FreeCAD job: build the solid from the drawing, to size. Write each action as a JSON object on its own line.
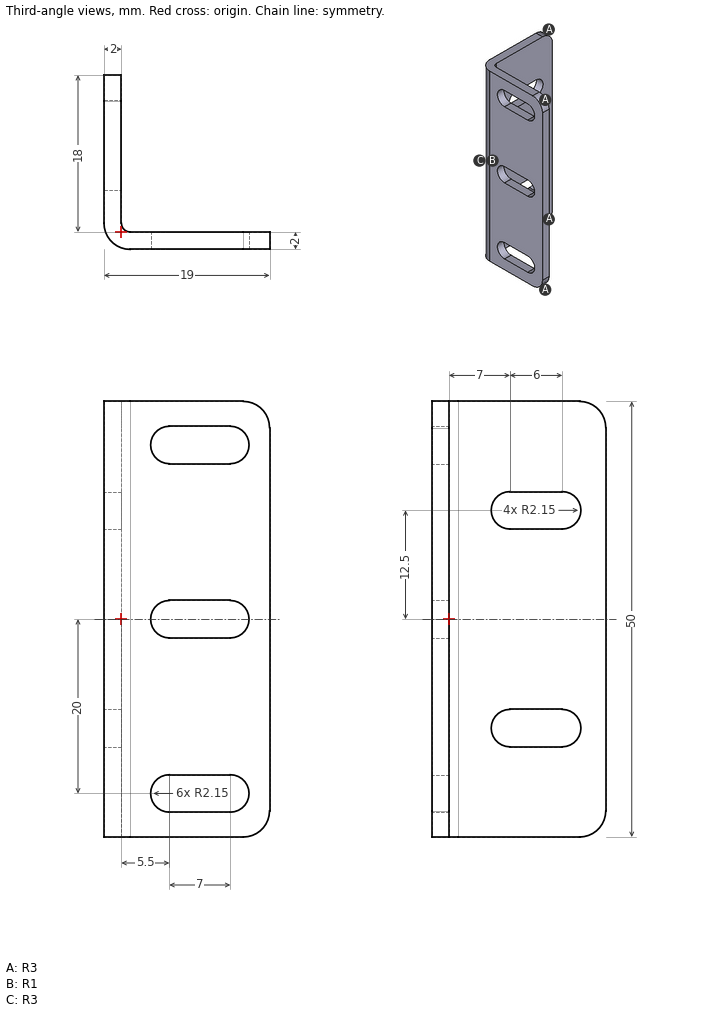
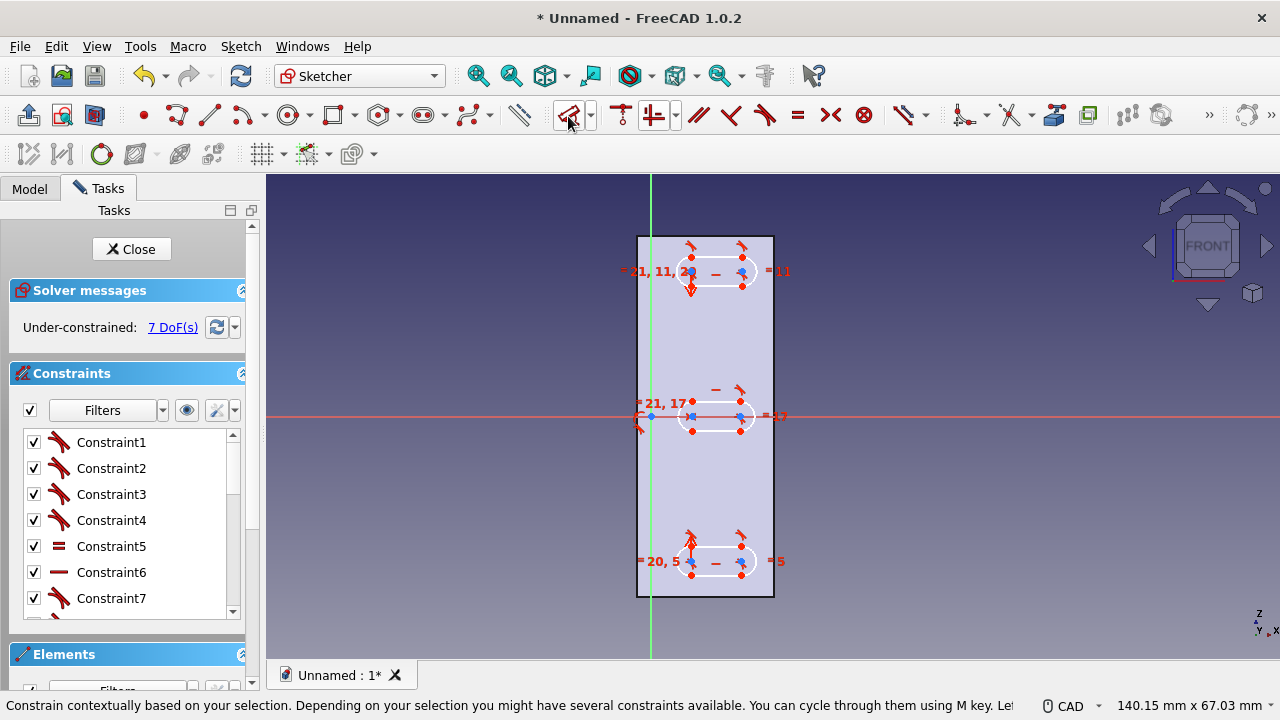
{"action": "scroll", "coordinate": [679, 553], "scroll_direction": "up", "scroll_amount": 5}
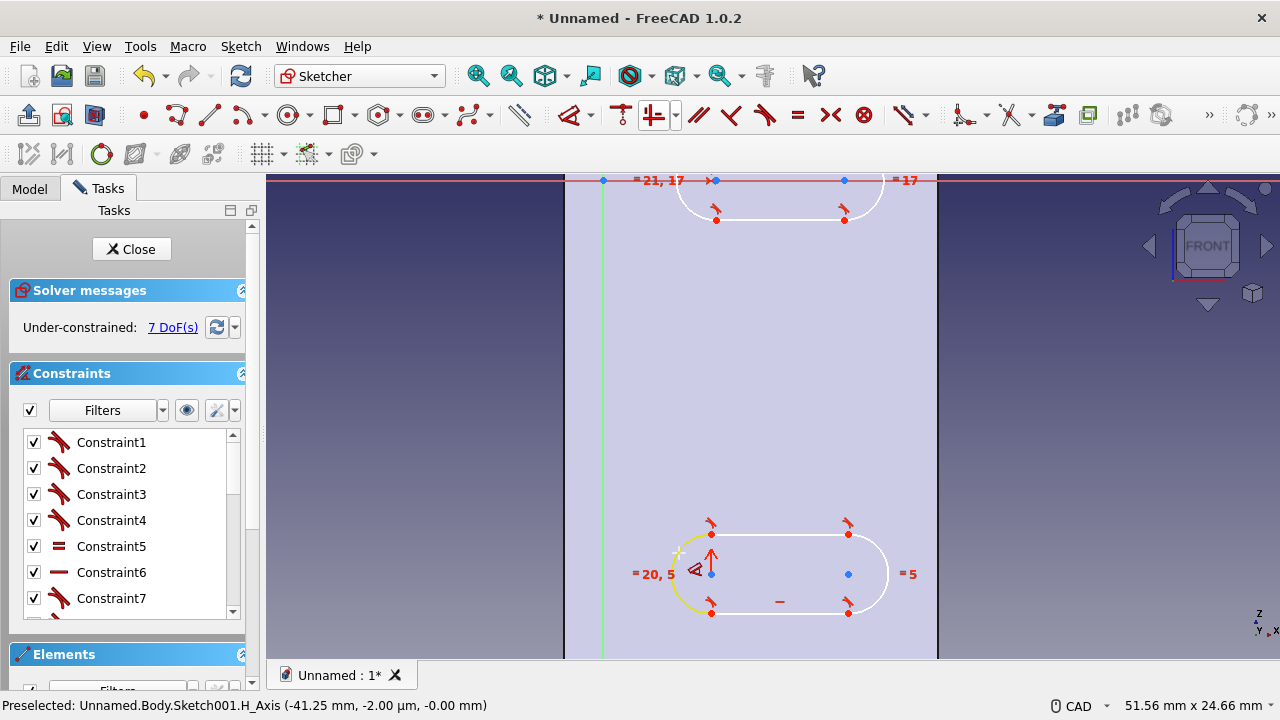
{"action": "left_click", "coordinate": [679, 551]}
{"action": "left_click", "coordinate": [653, 532]}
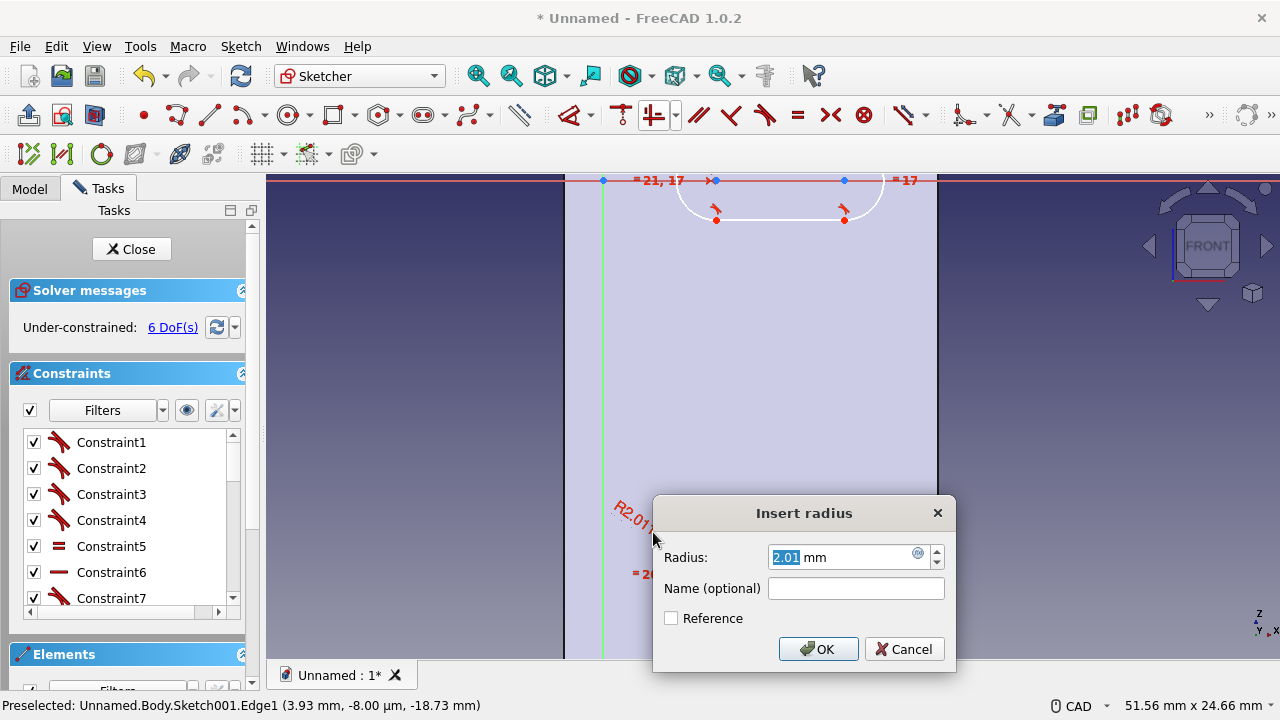
{"action": "type", "text": "2.15"}
{"action": "key", "text": "Return"}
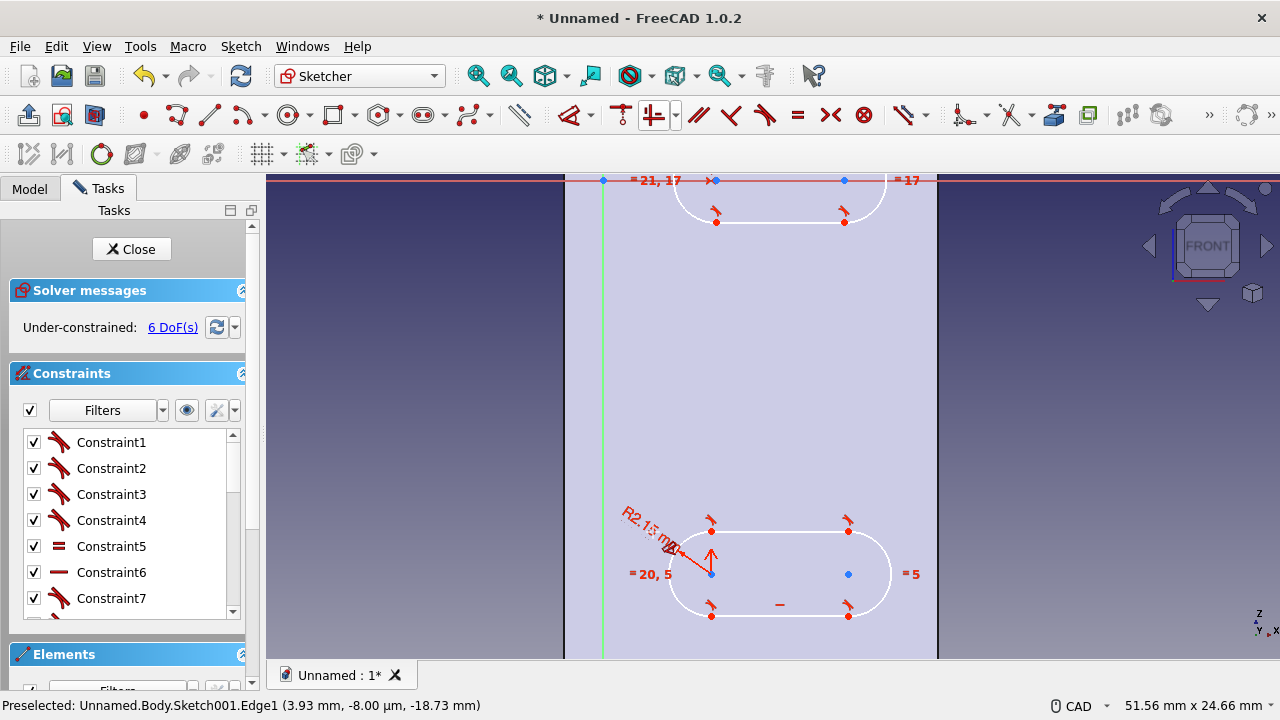
{"action": "left_click", "coordinate": [753, 532]}
{"action": "left_click", "coordinate": [780, 566]}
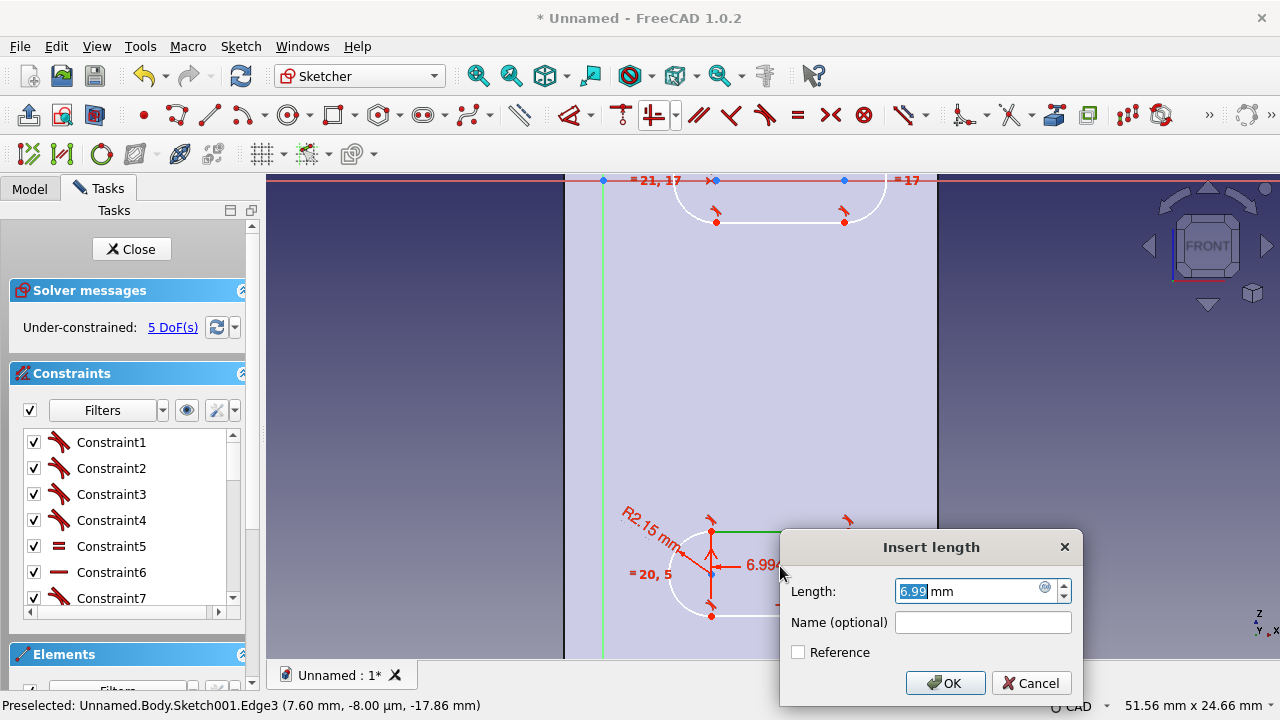
{"action": "type", "text": "7"}
{"action": "key", "text": "Return"}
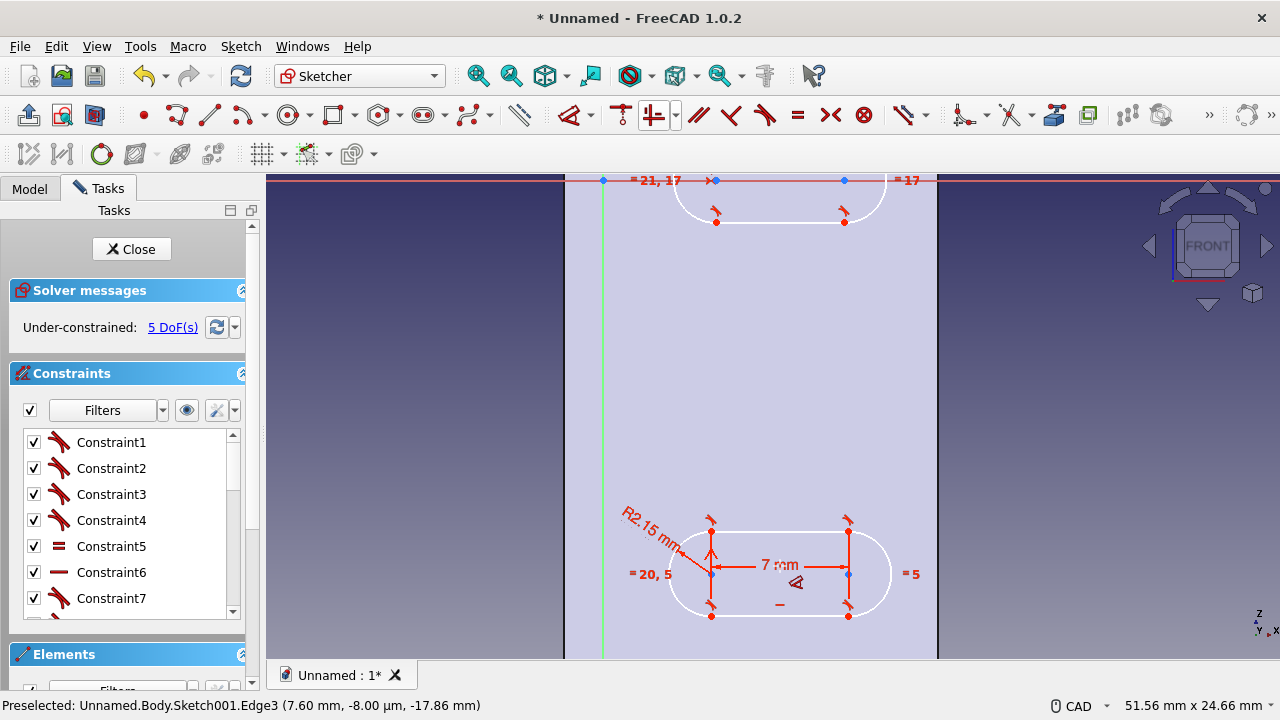
{"action": "scroll", "coordinate": [679, 554], "scroll_direction": "down", "scroll_amount": 5}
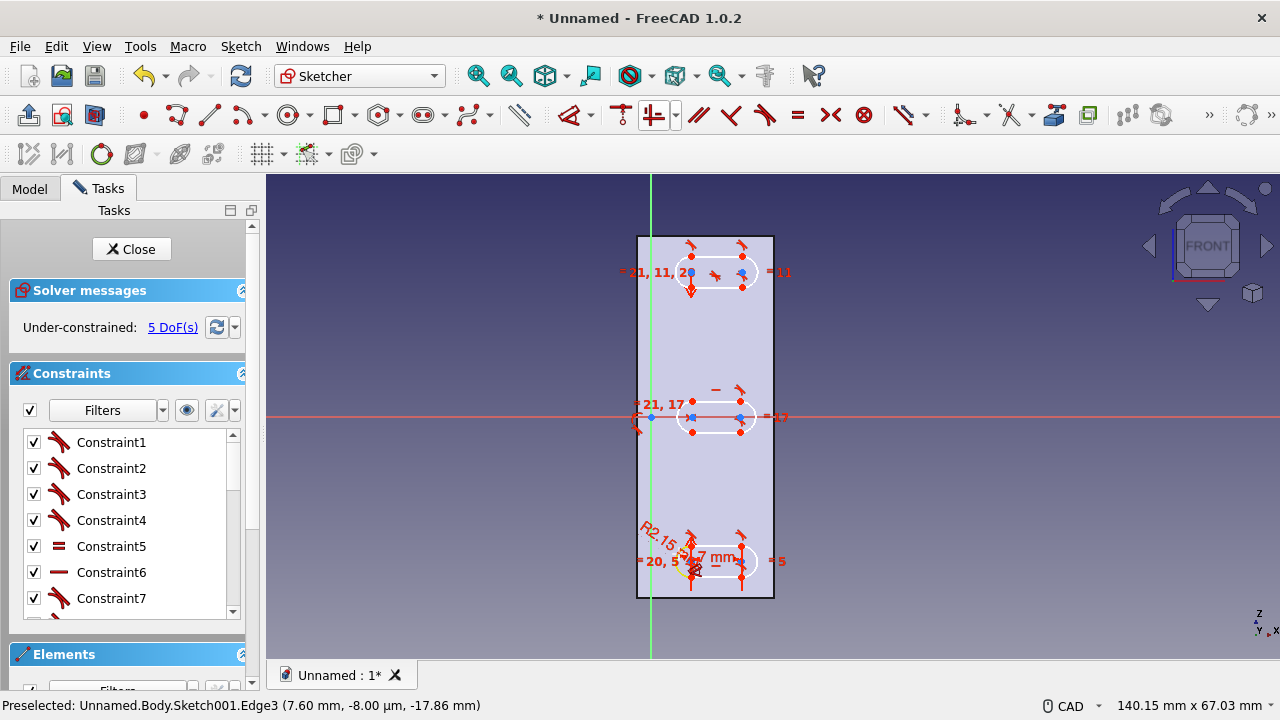
{"action": "left_click", "coordinate": [706, 257]}
{"action": "left_click", "coordinate": [717, 223]}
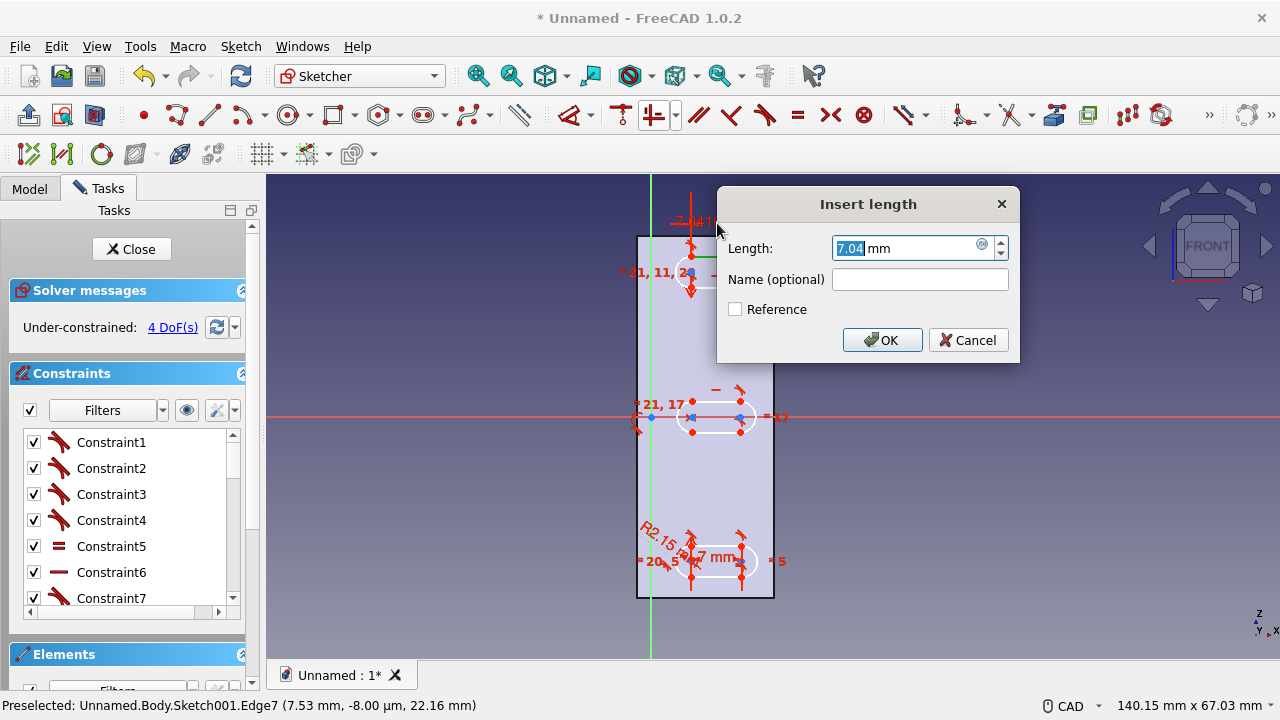
{"action": "type", "text": "7"}
{"action": "key", "text": "Return"}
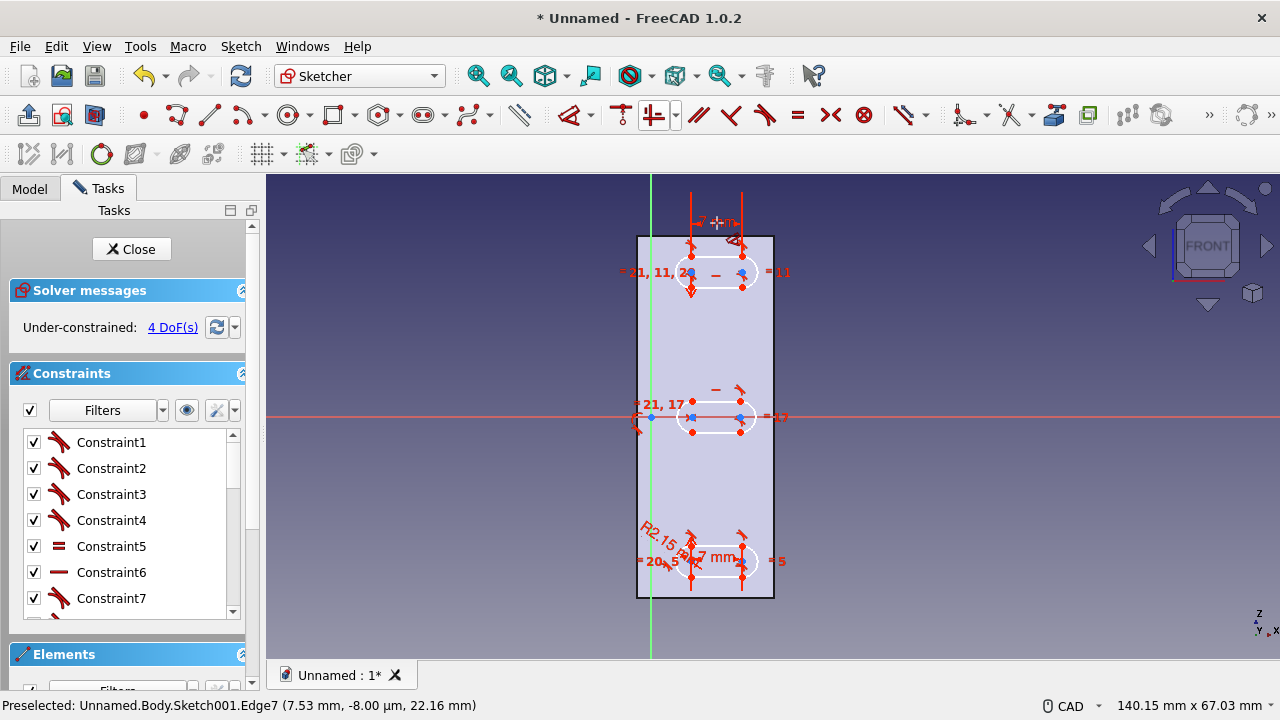
{"action": "left_click", "coordinate": [707, 402]}
{"action": "left_click", "coordinate": [716, 368]}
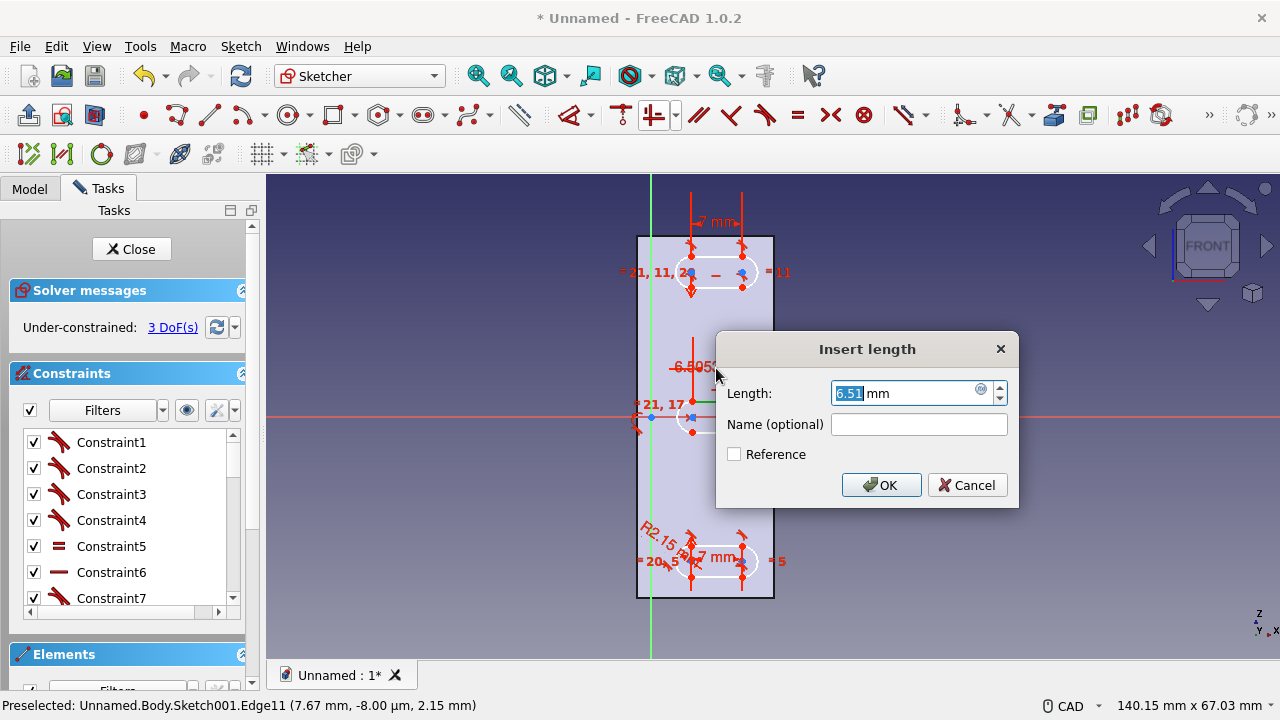
{"action": "type", "text": "7"}
{"action": "key", "text": "Return"}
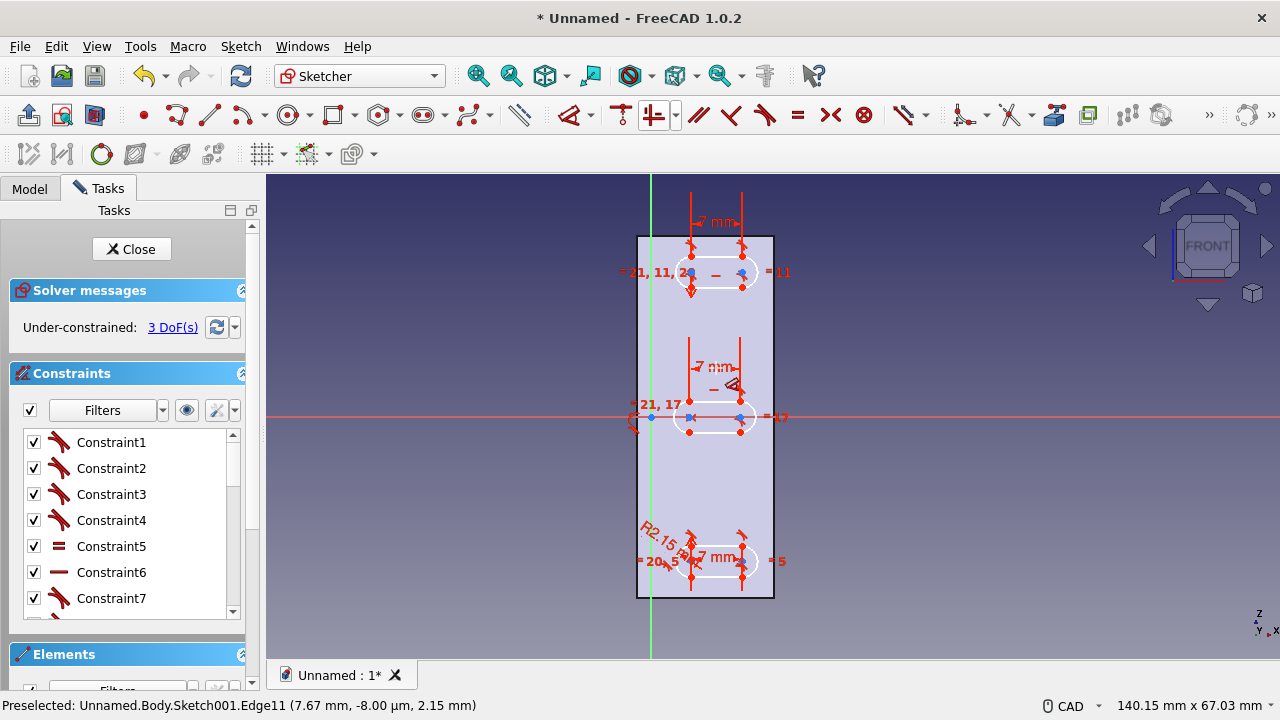
{"action": "left_click", "coordinate": [691, 562]}
{"action": "left_click", "coordinate": [617, 490]}